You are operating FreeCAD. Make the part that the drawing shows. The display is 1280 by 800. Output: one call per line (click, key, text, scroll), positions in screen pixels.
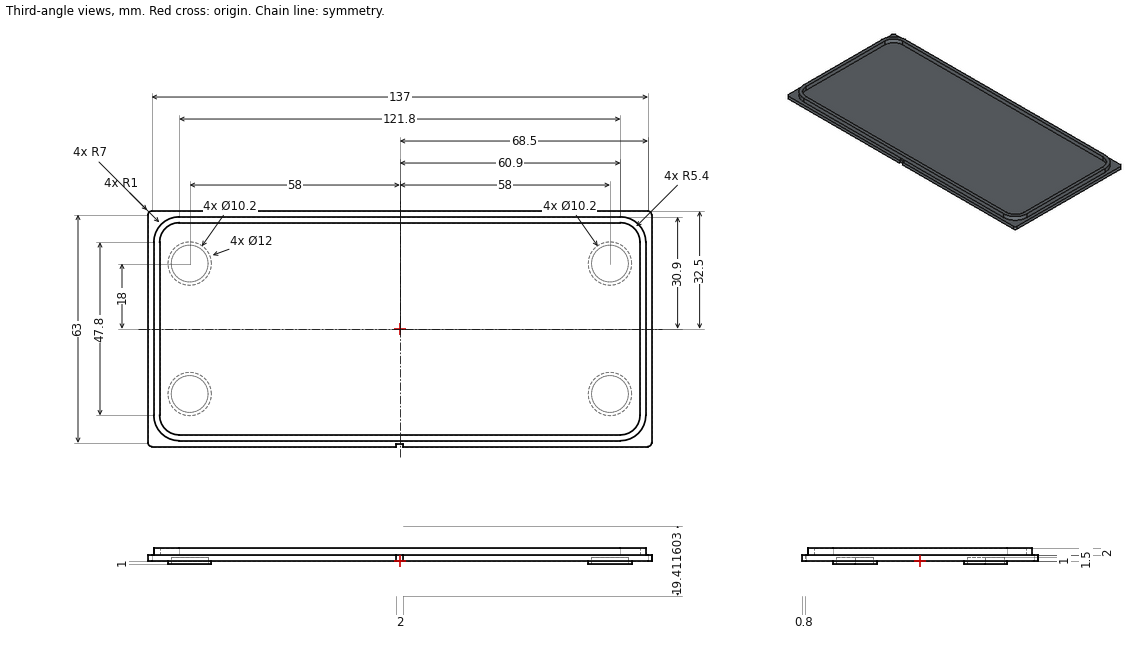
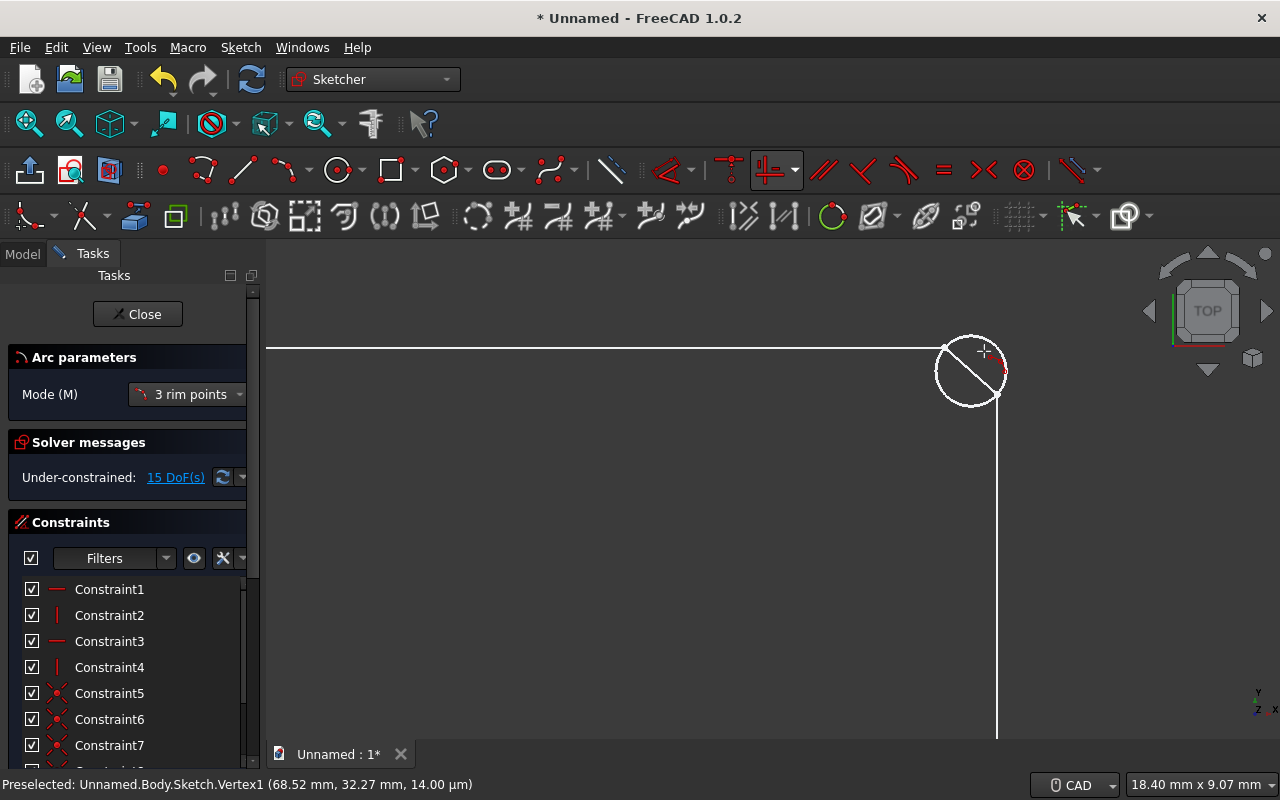
click(983, 351)
key(Escape)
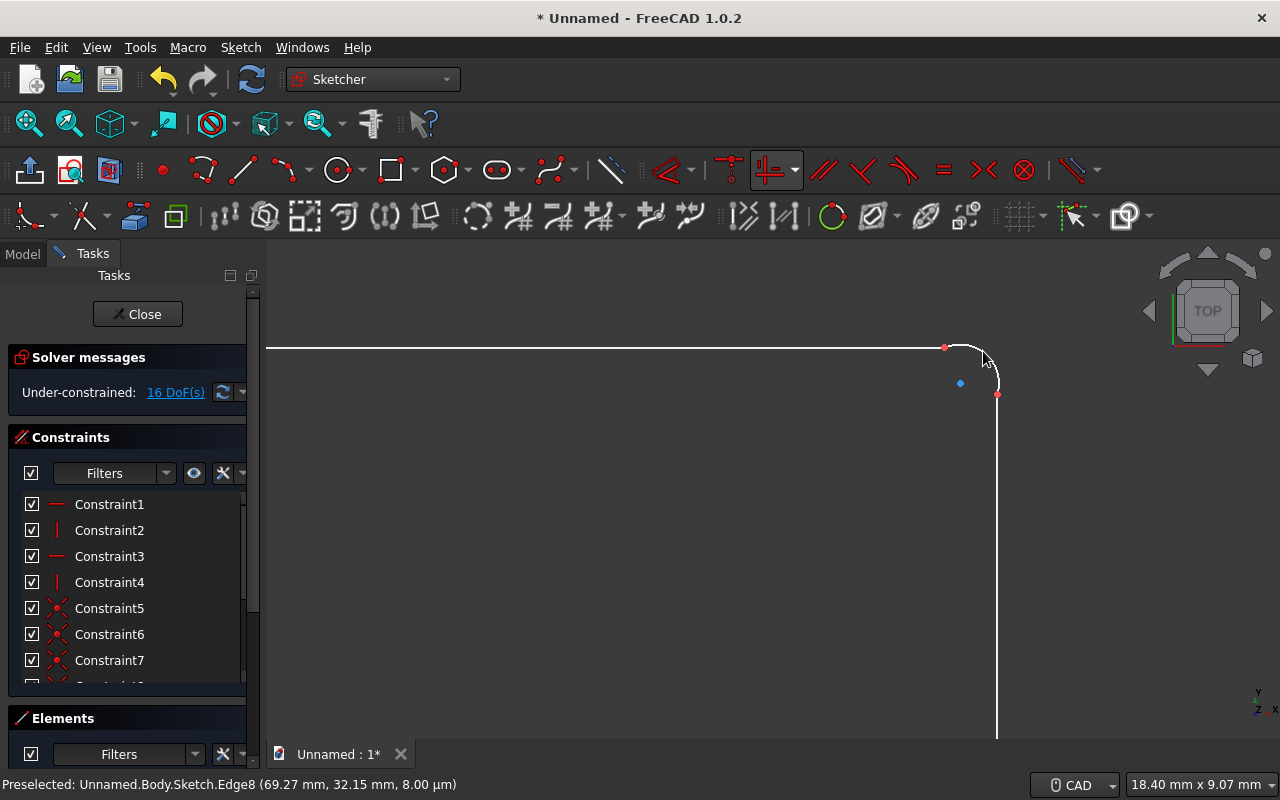
scroll(988, 358, down, 13)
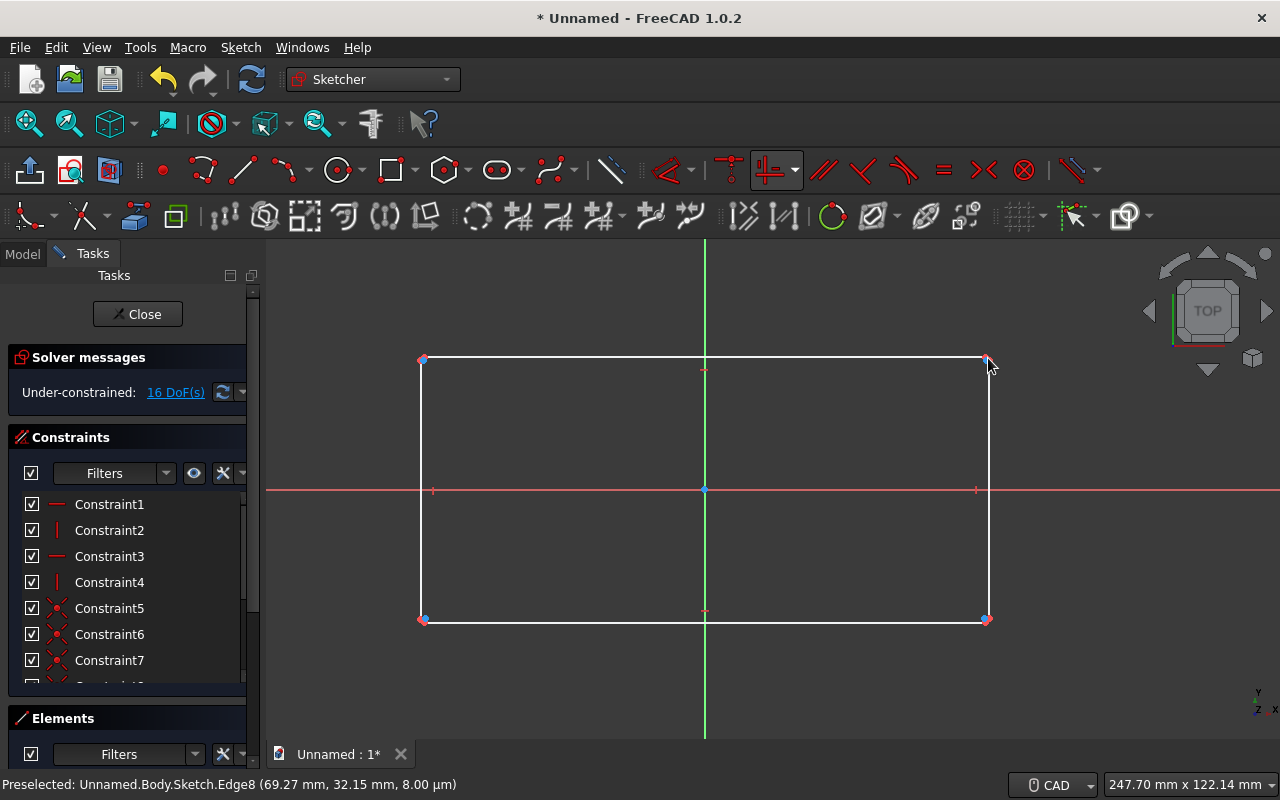
click(817, 357)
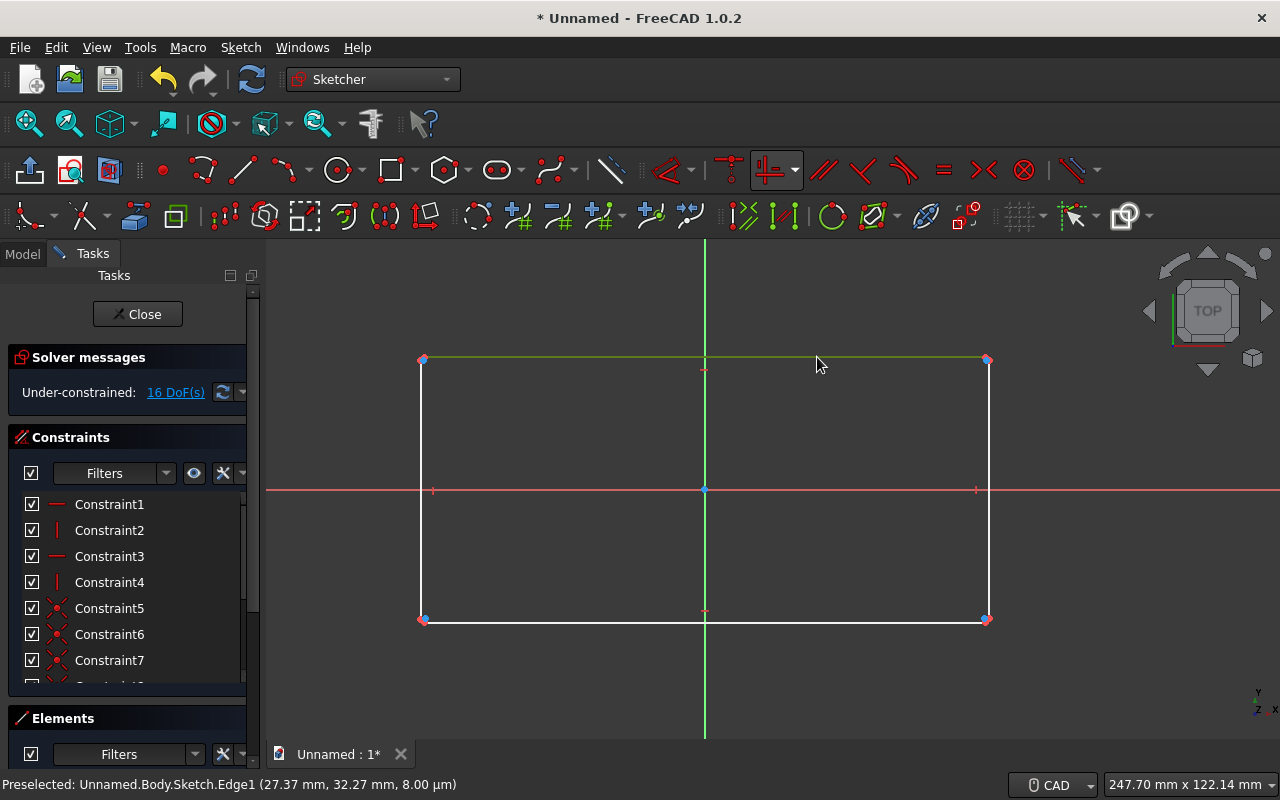
scroll(421, 358, up, 8)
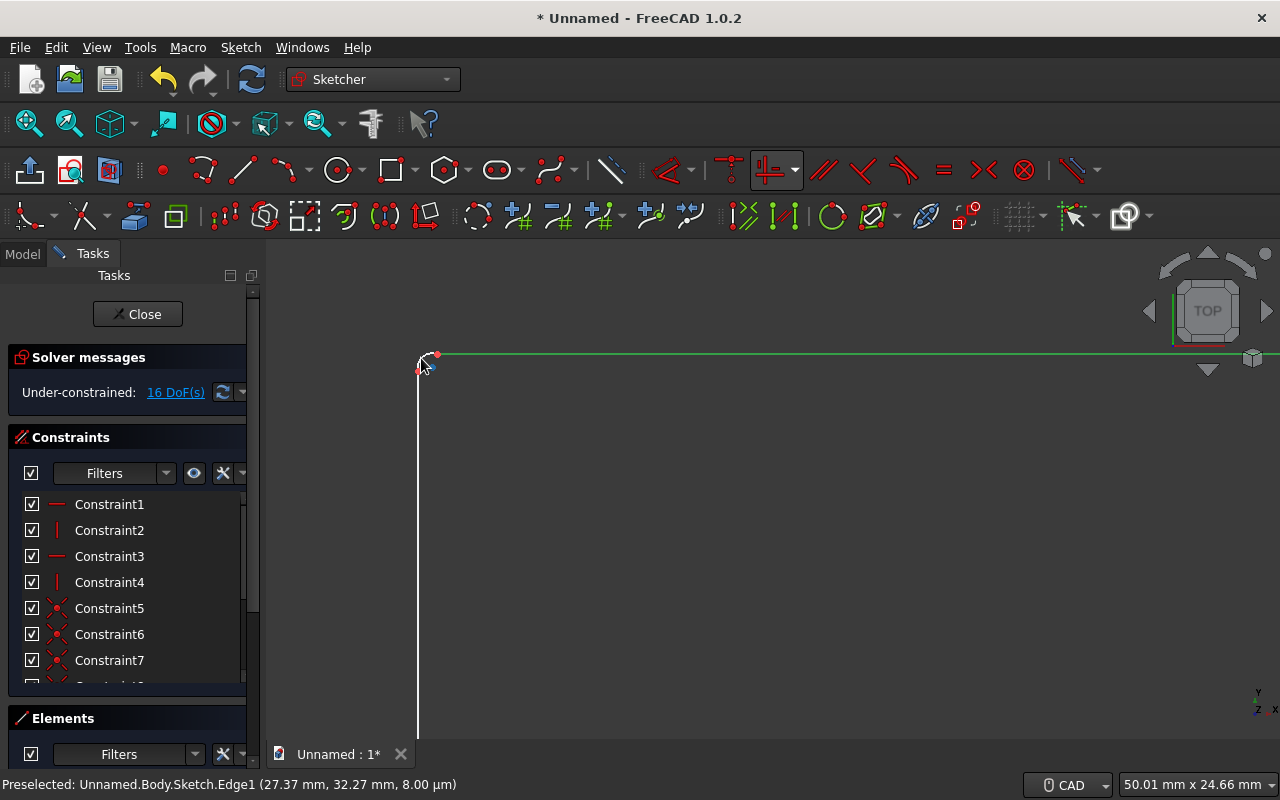
click(423, 357)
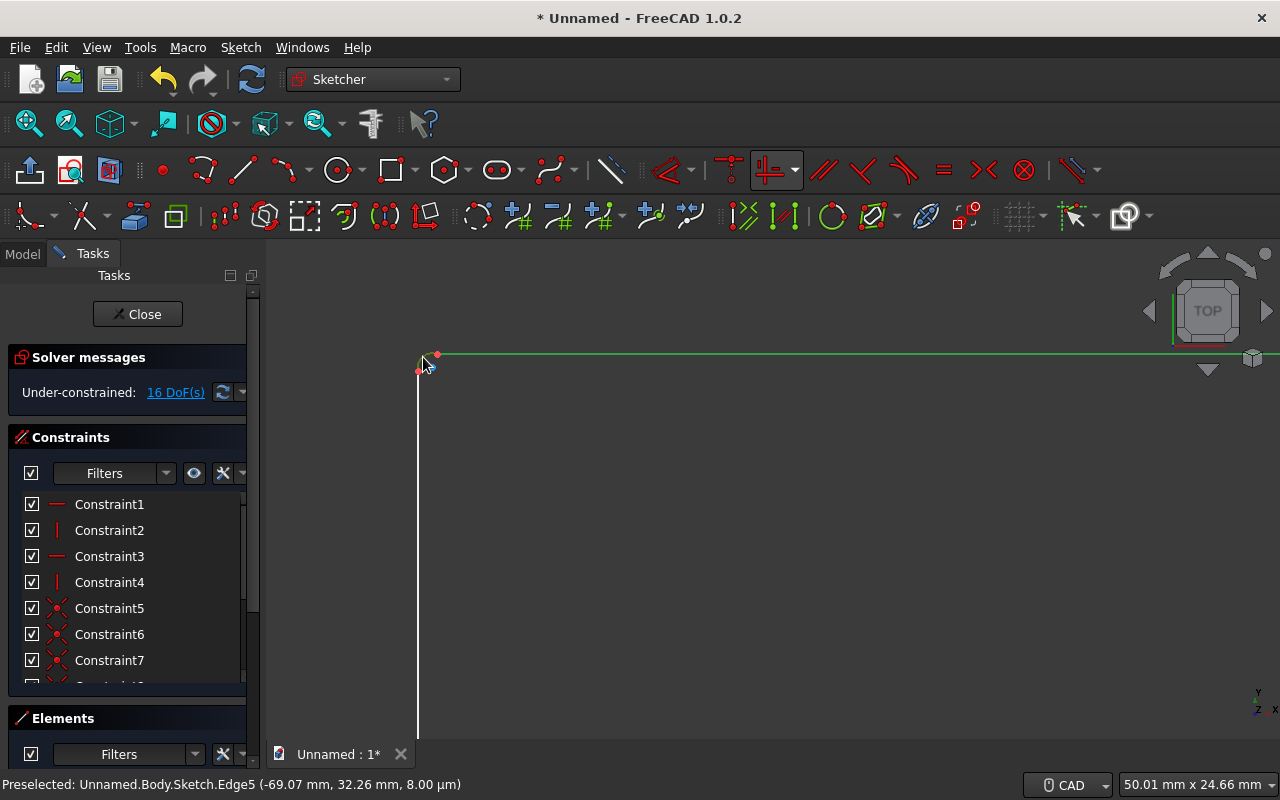
click(904, 170)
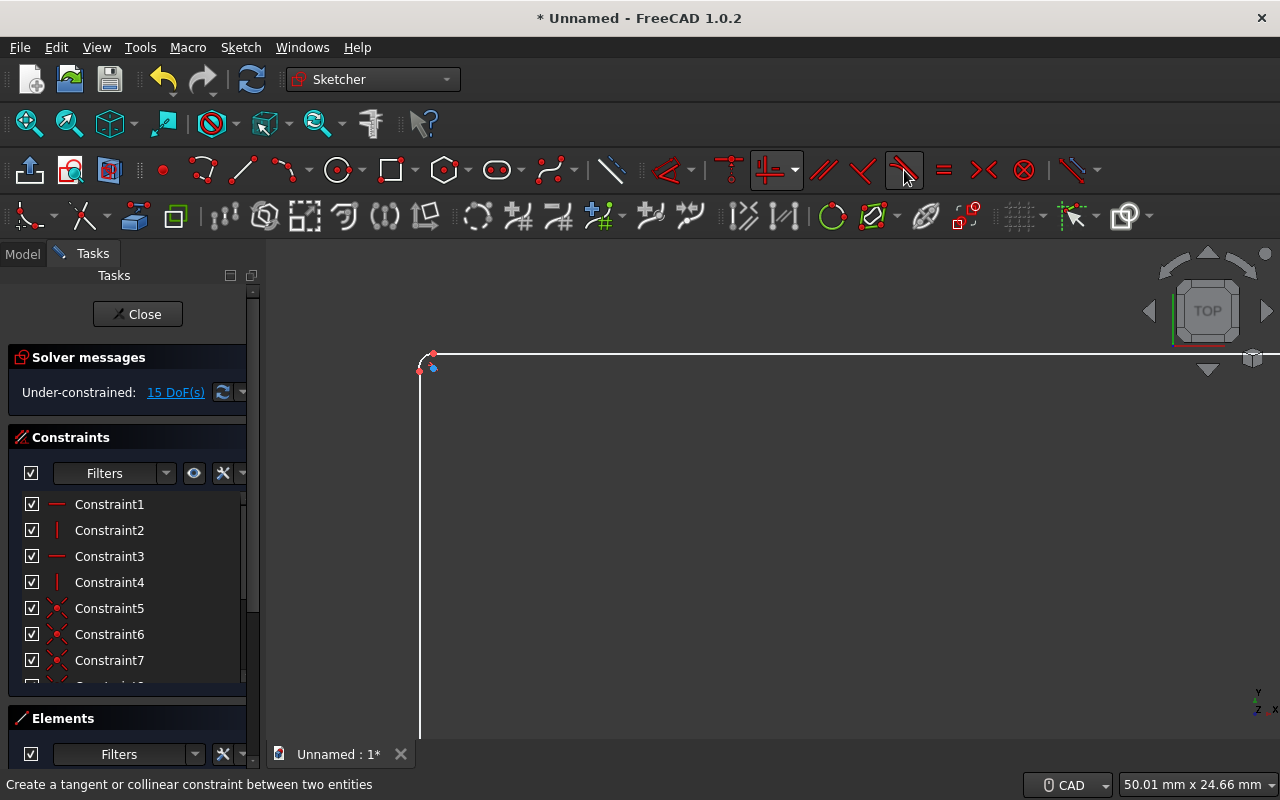
scroll(421, 358, down, 8)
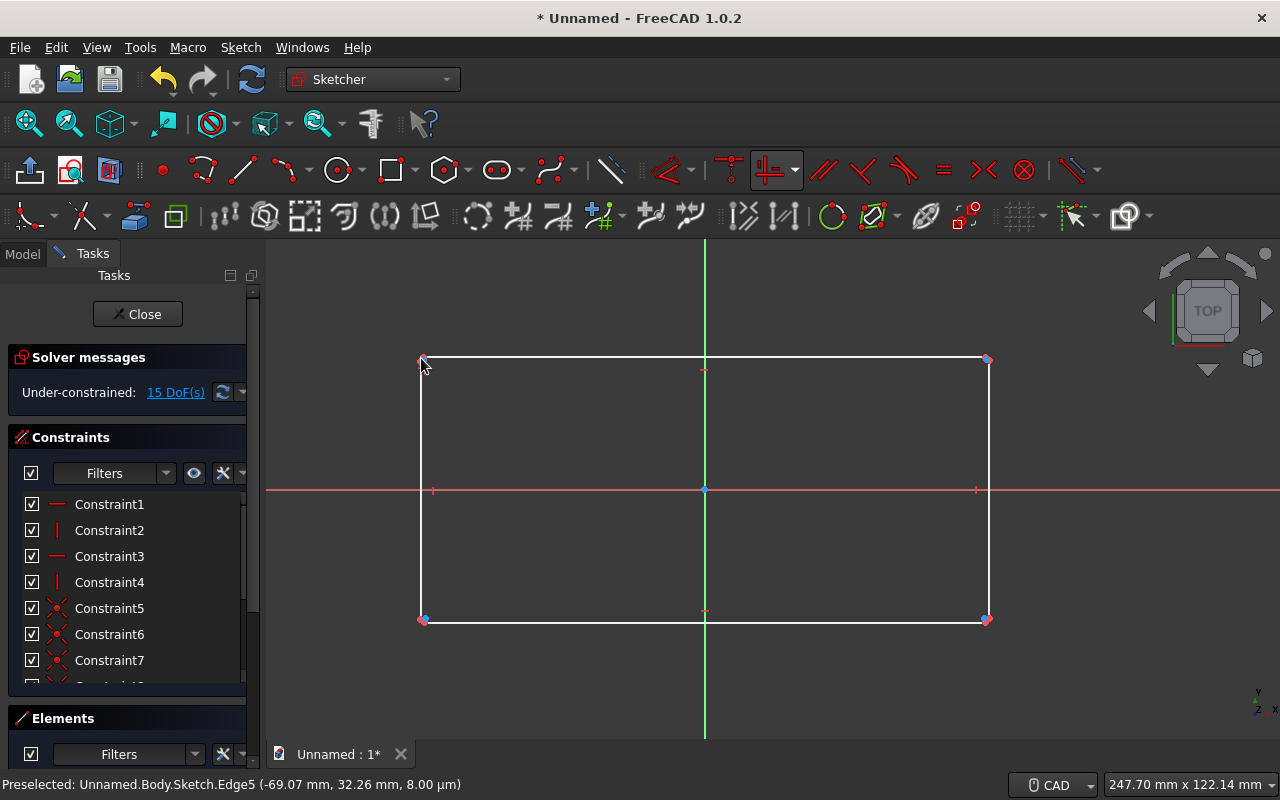
click(536, 357)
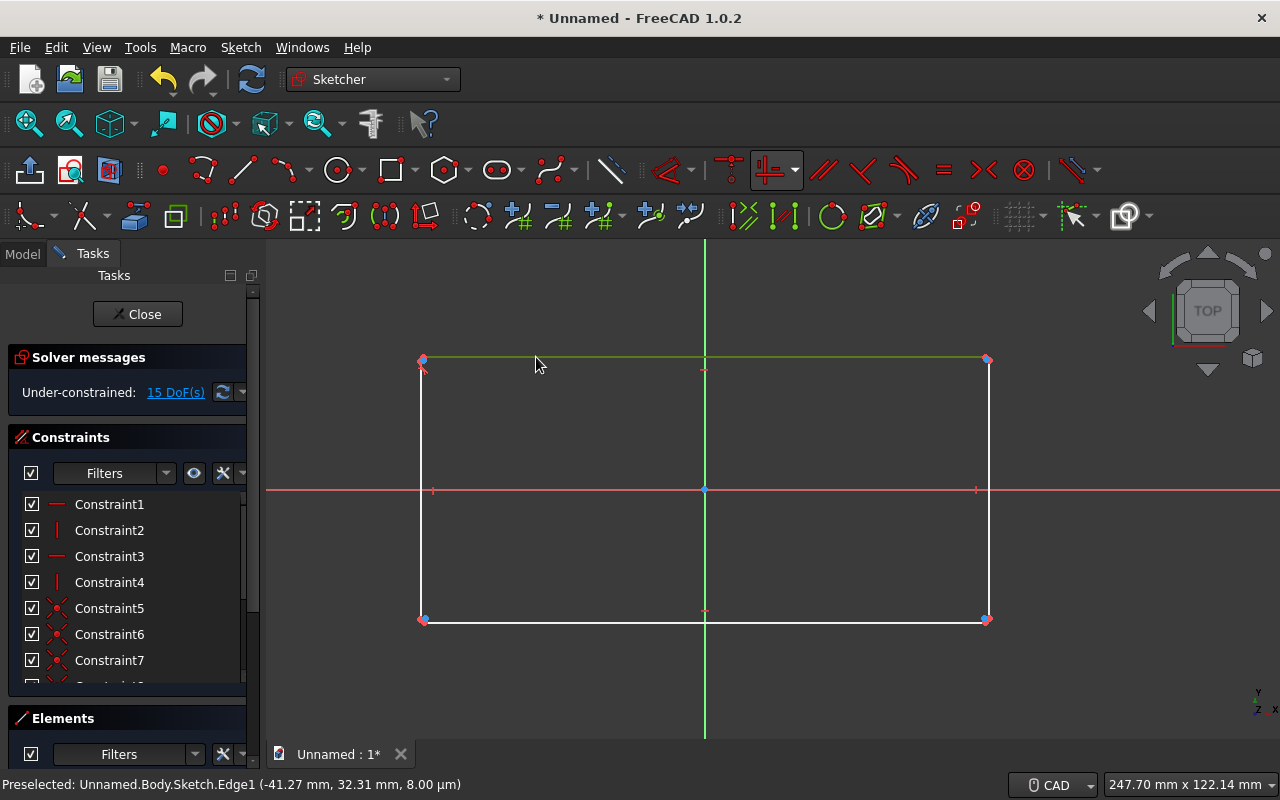
scroll(988, 358, up, 9)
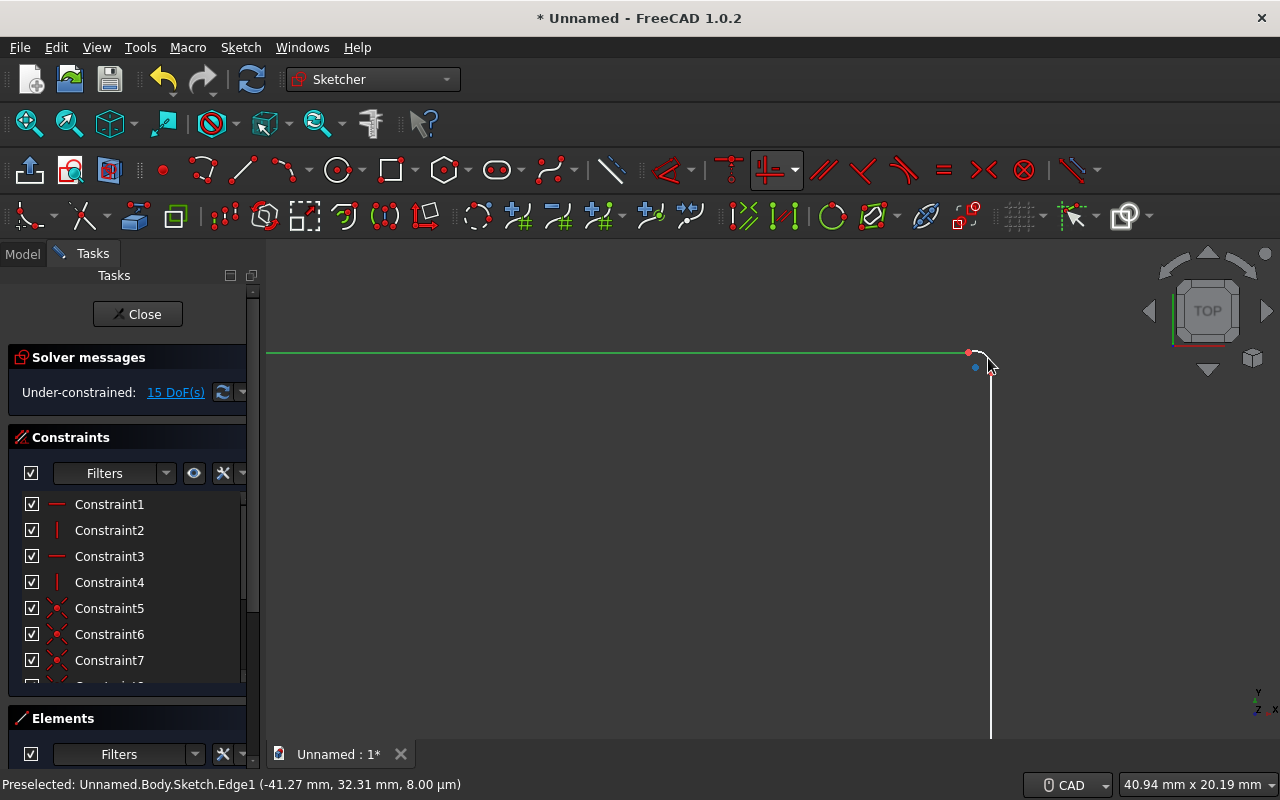
click(986, 355)